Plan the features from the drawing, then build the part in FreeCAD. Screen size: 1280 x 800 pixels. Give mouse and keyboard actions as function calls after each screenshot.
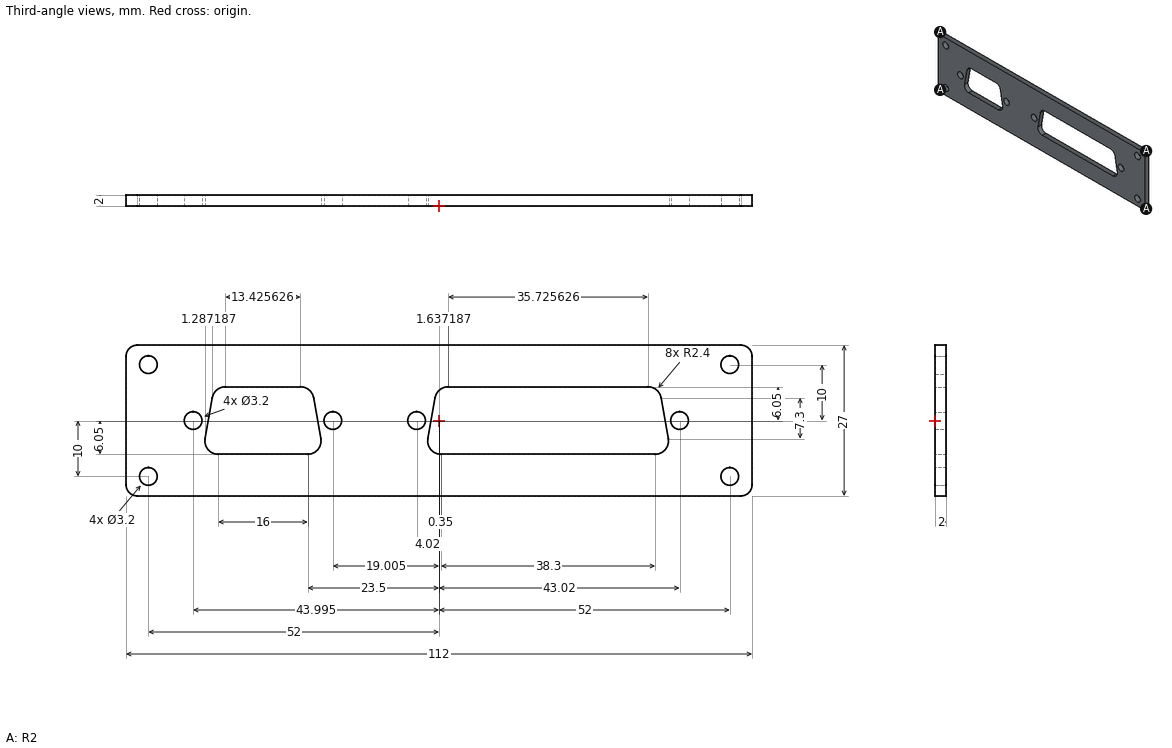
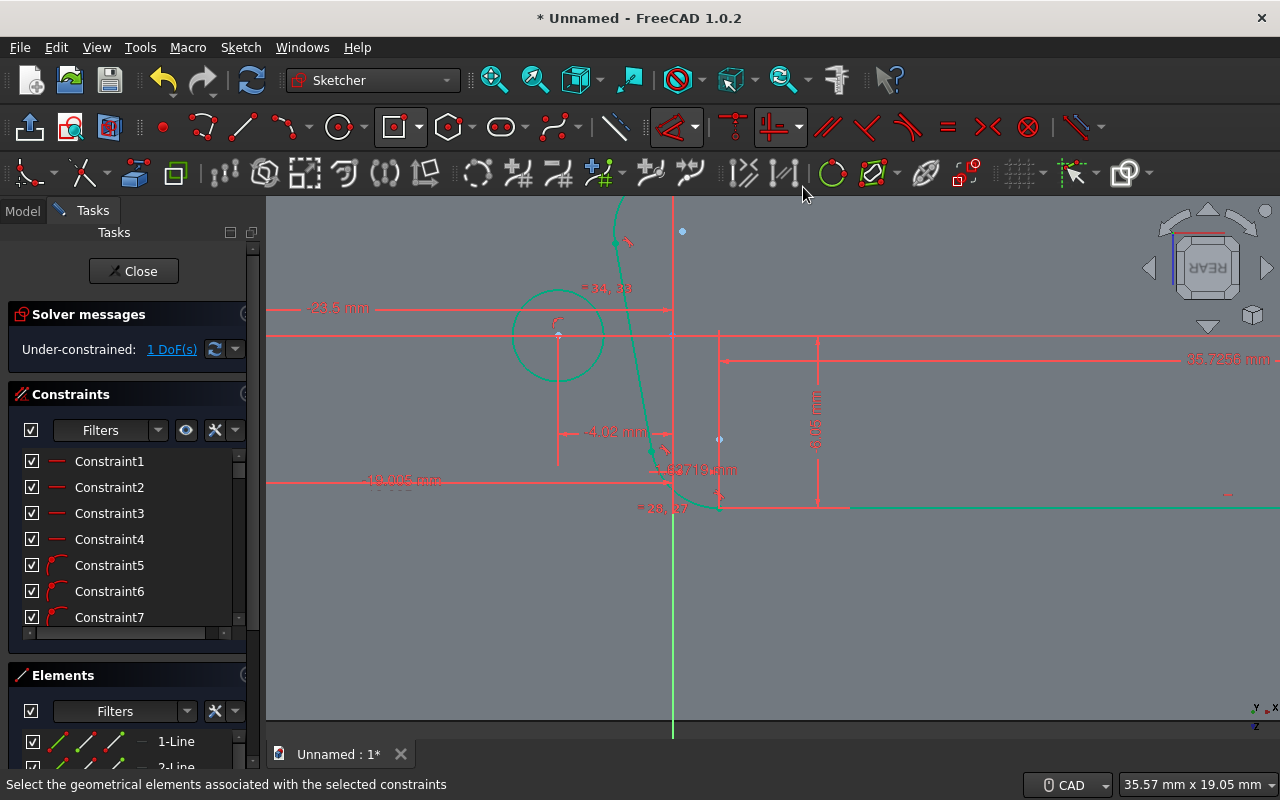
scroll(719, 511, down, 7)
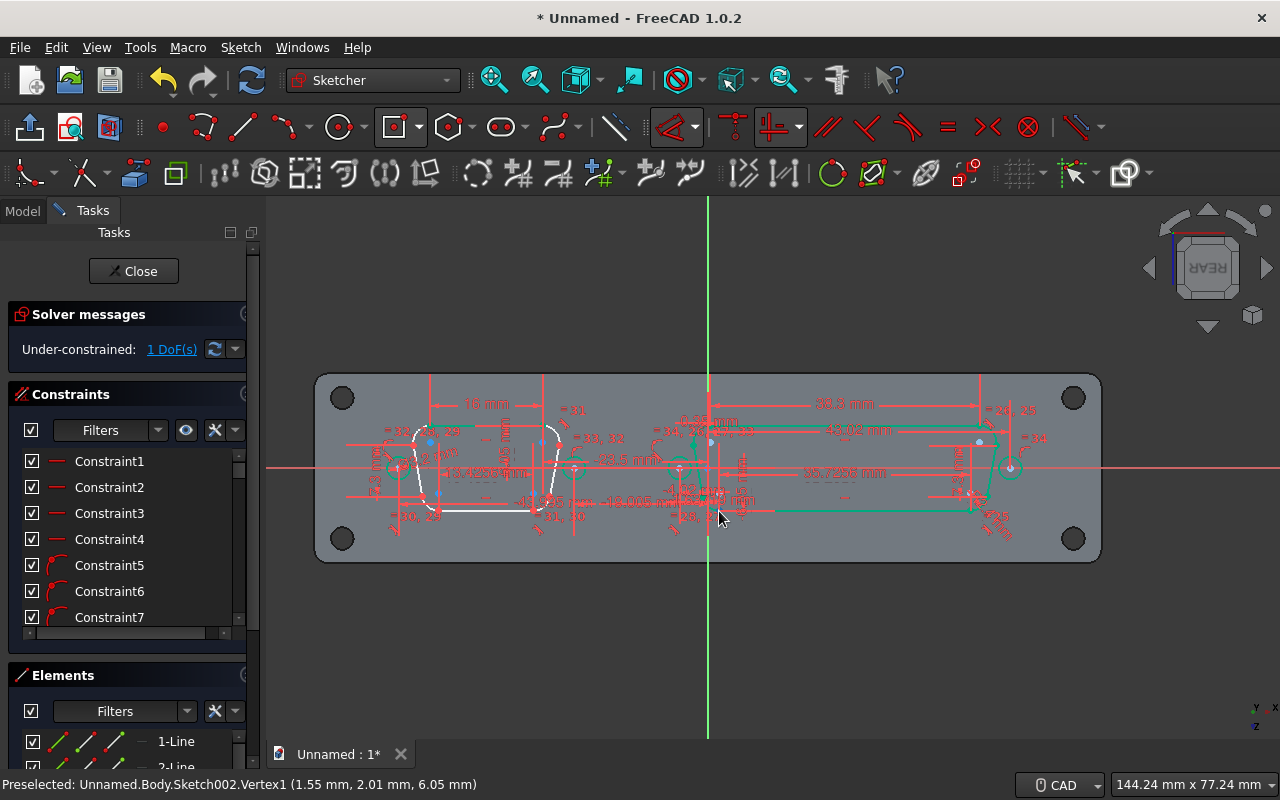
scroll(416, 461, up, 8)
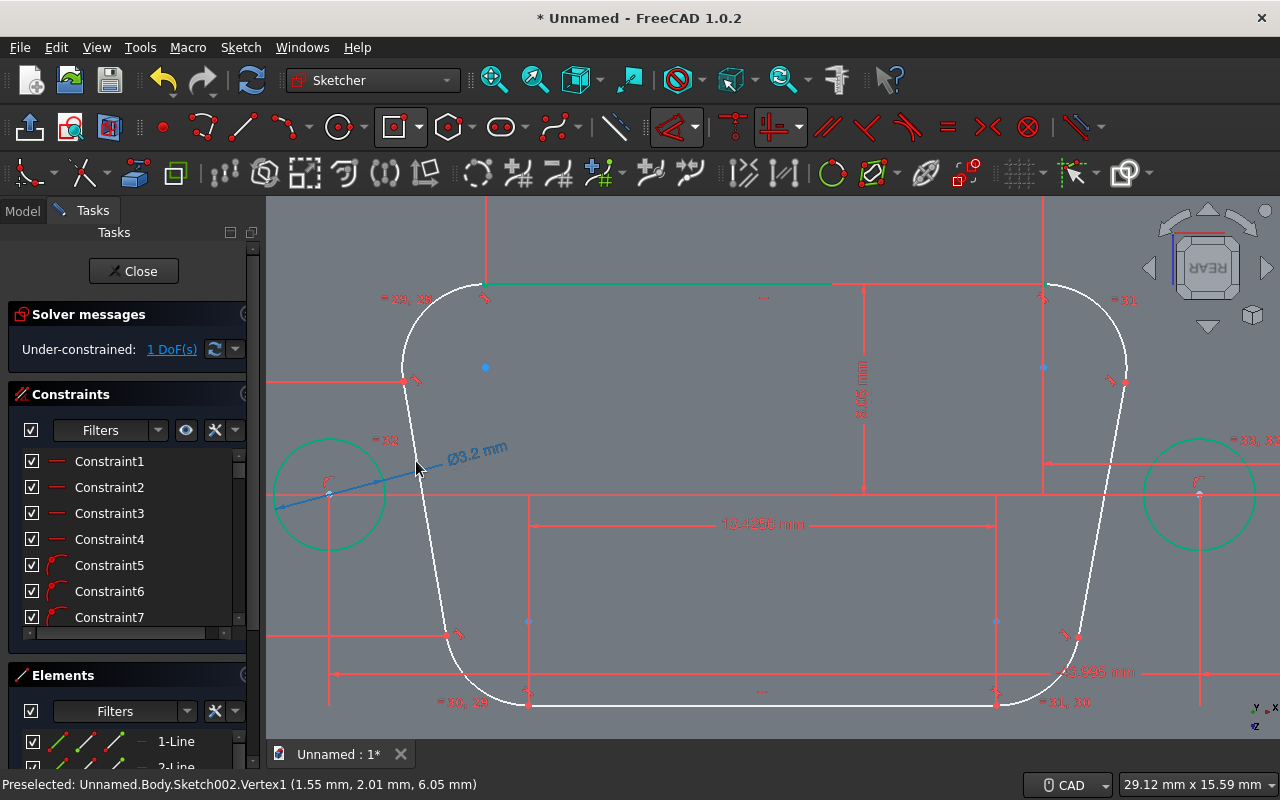
click(416, 458)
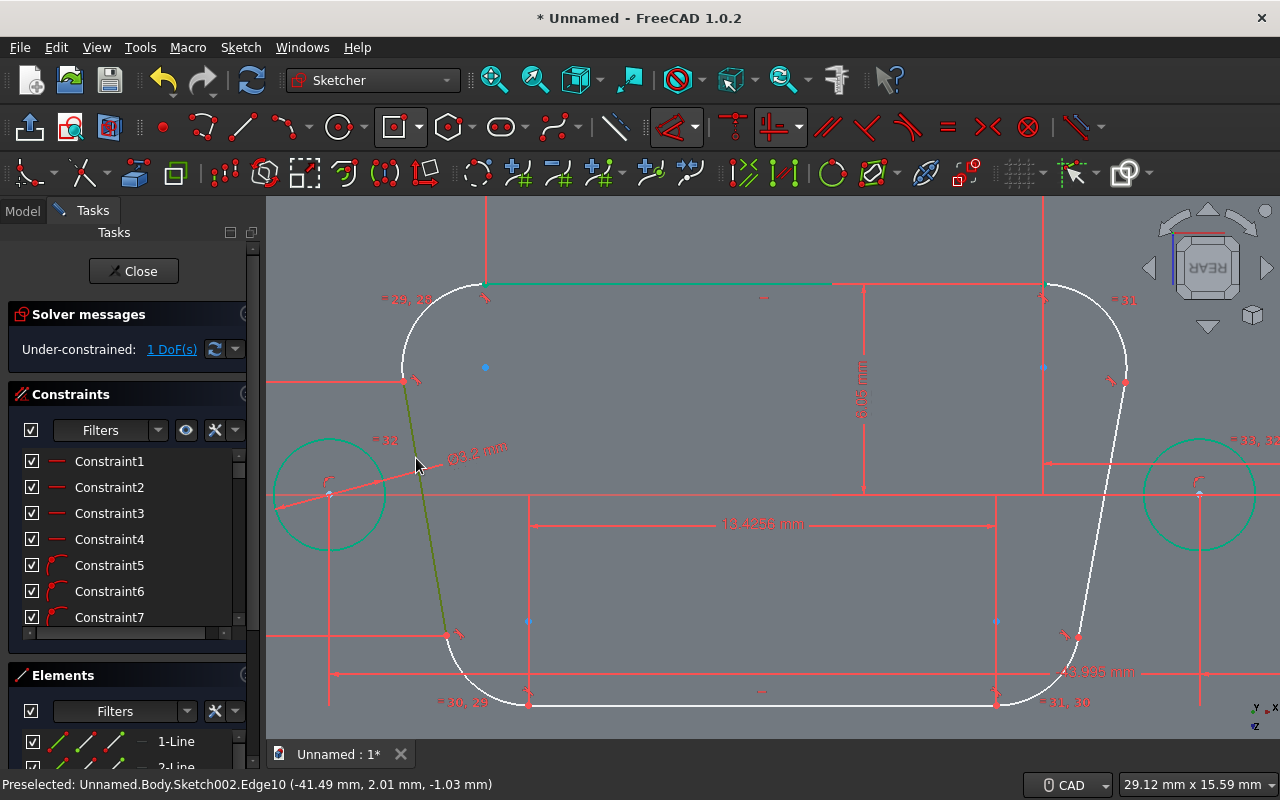
click(698, 128)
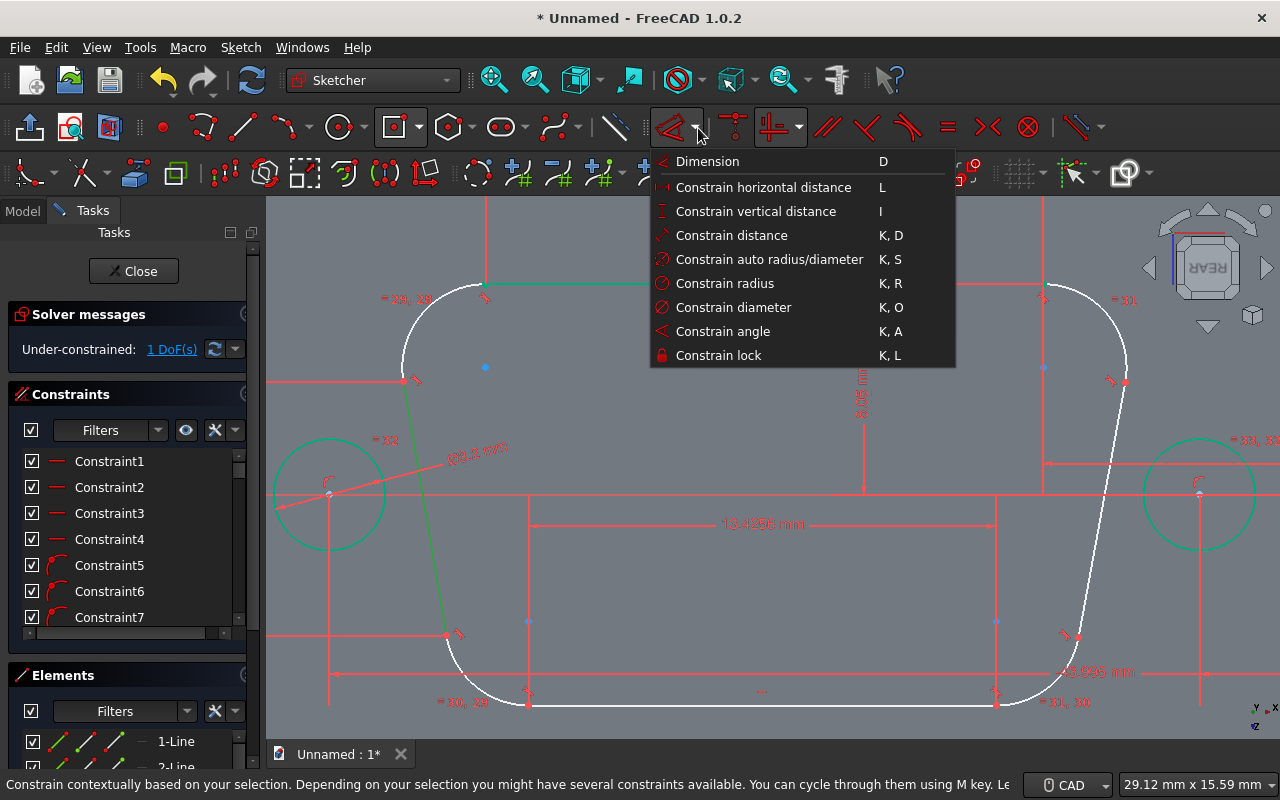
click(803, 187)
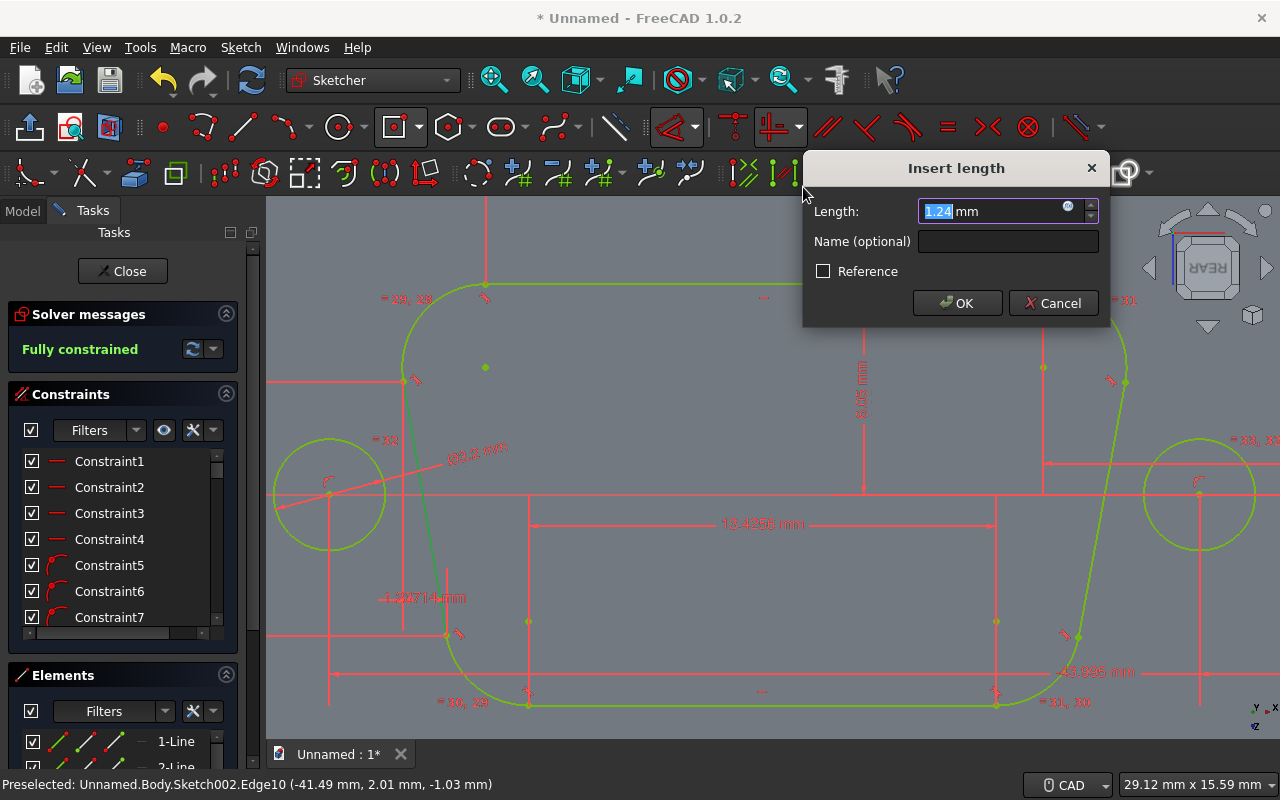
text(1.287187)
key(Return)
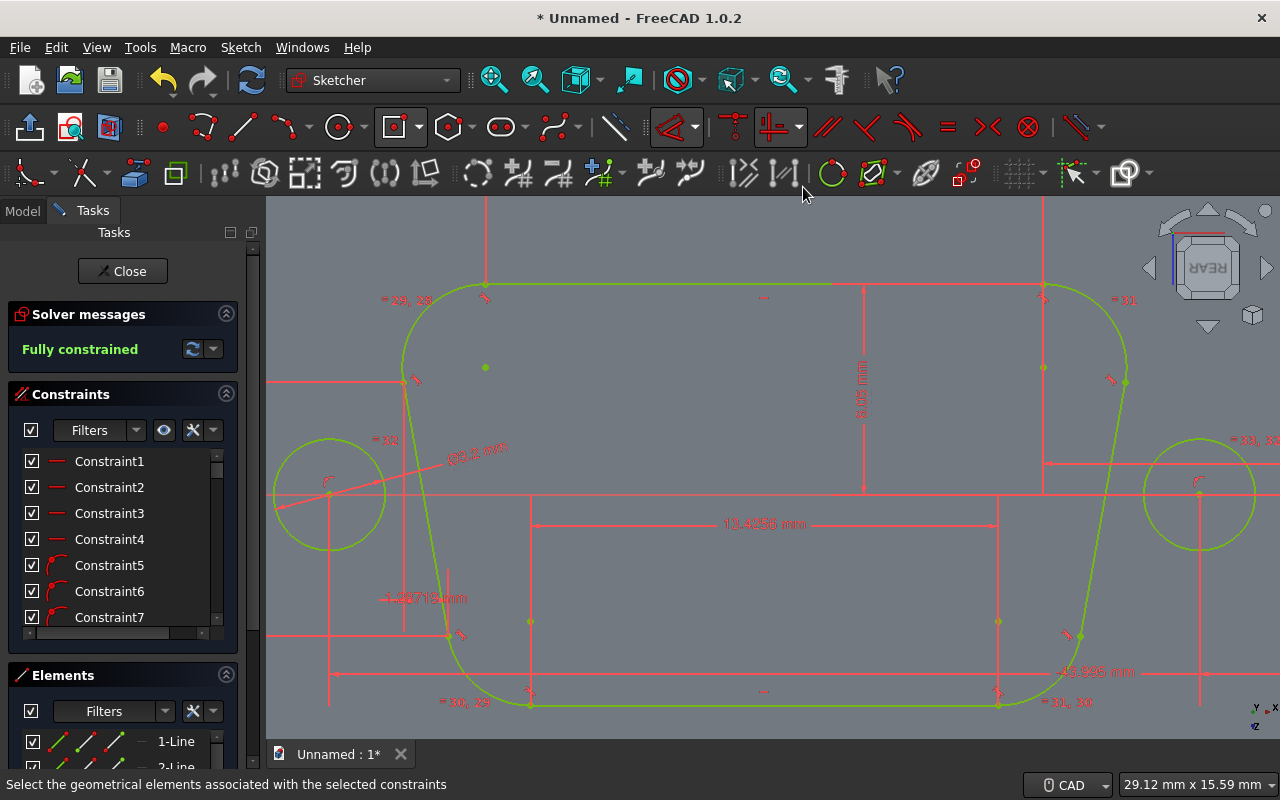
click(123, 271)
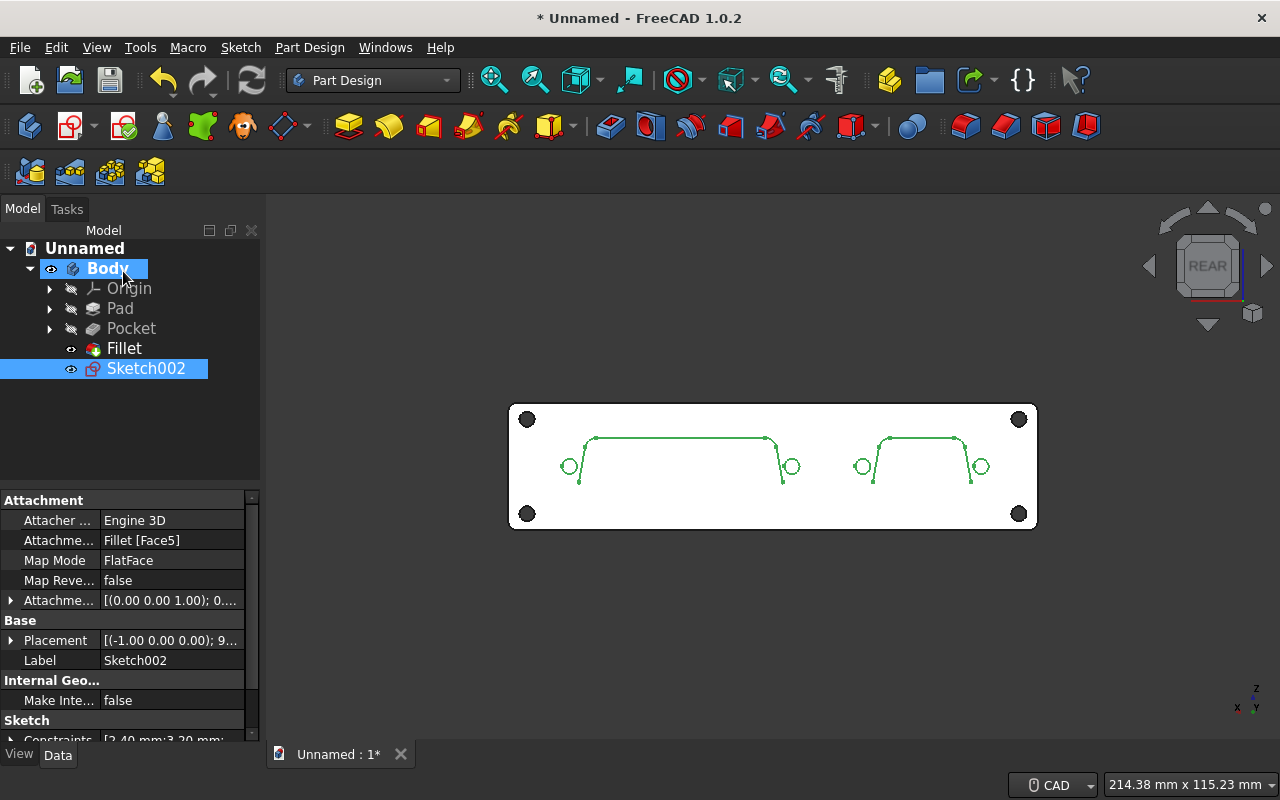
click(612, 126)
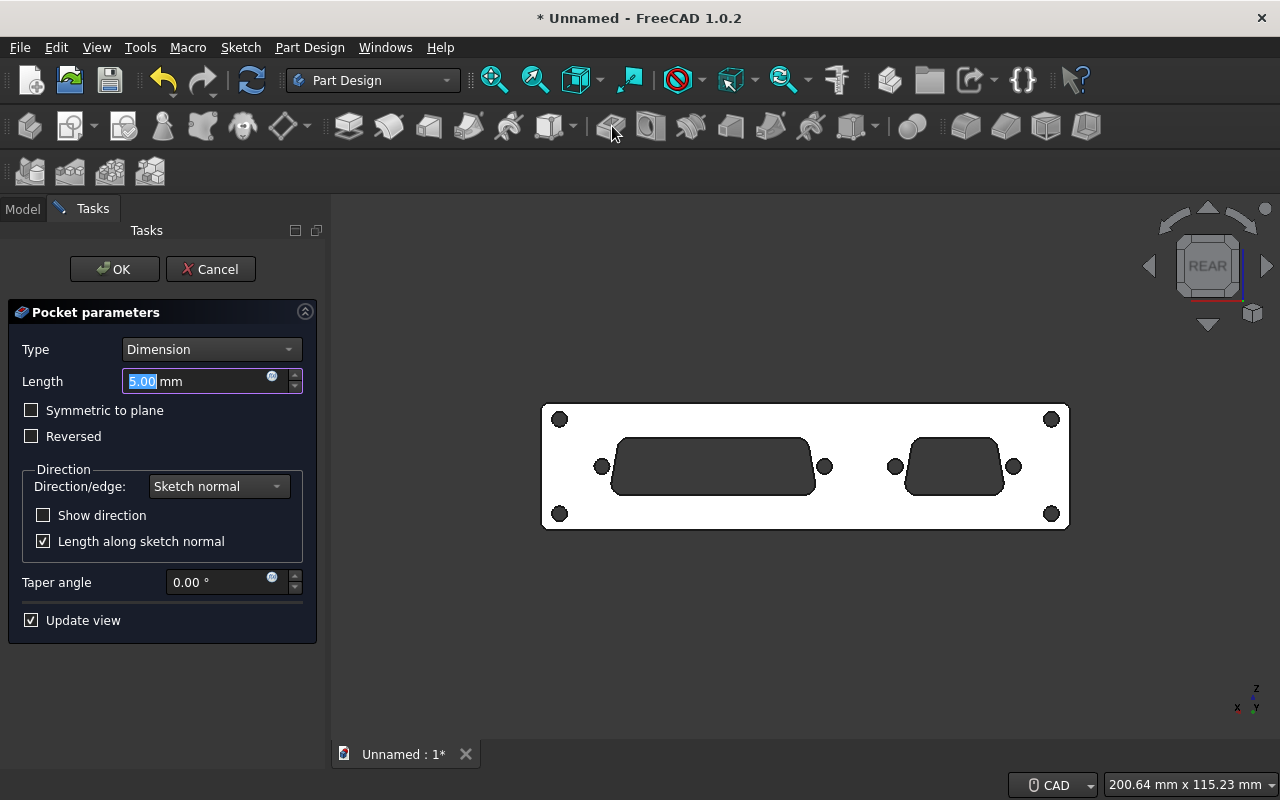
text(2)
key(Tab)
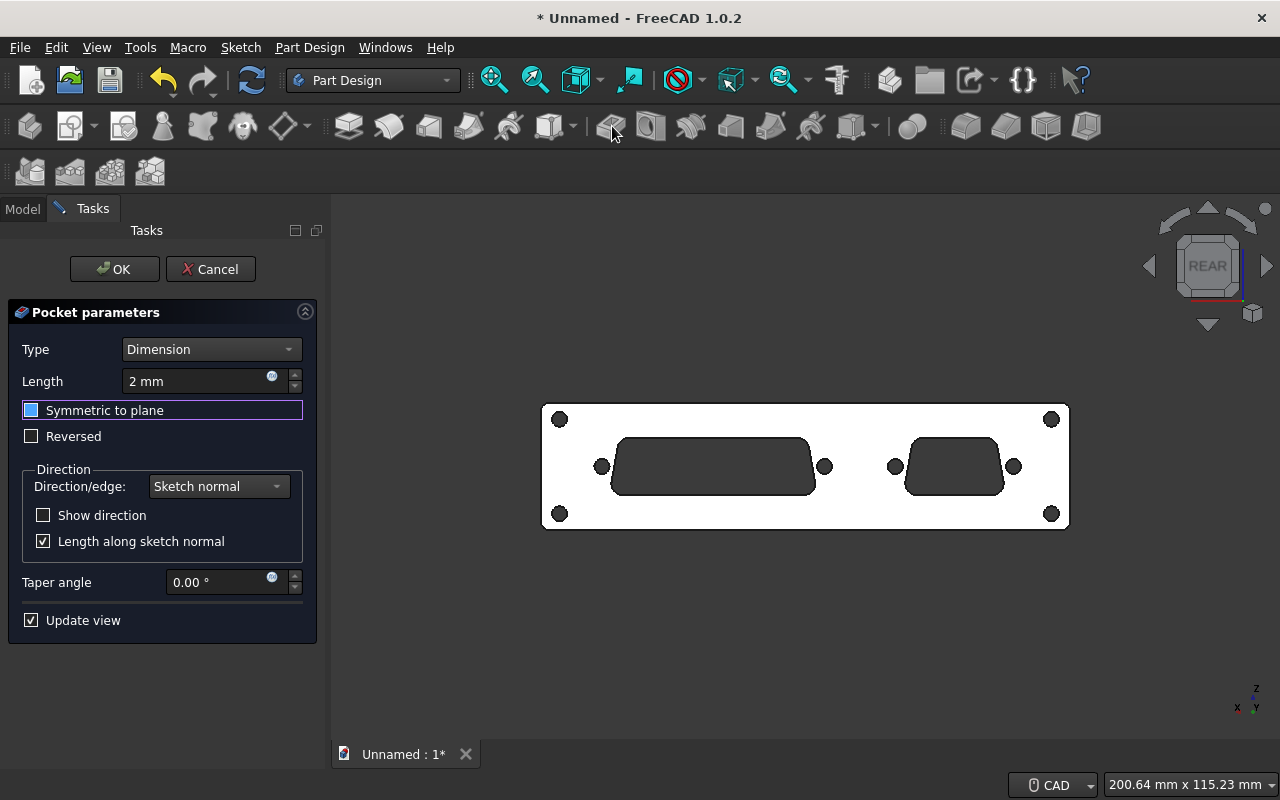
click(115, 269)